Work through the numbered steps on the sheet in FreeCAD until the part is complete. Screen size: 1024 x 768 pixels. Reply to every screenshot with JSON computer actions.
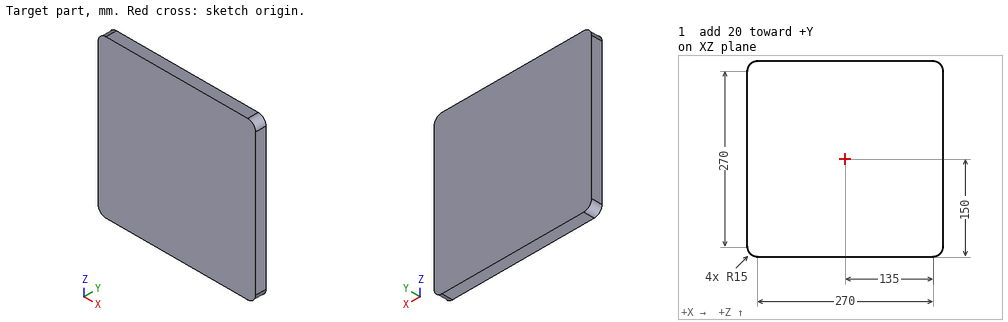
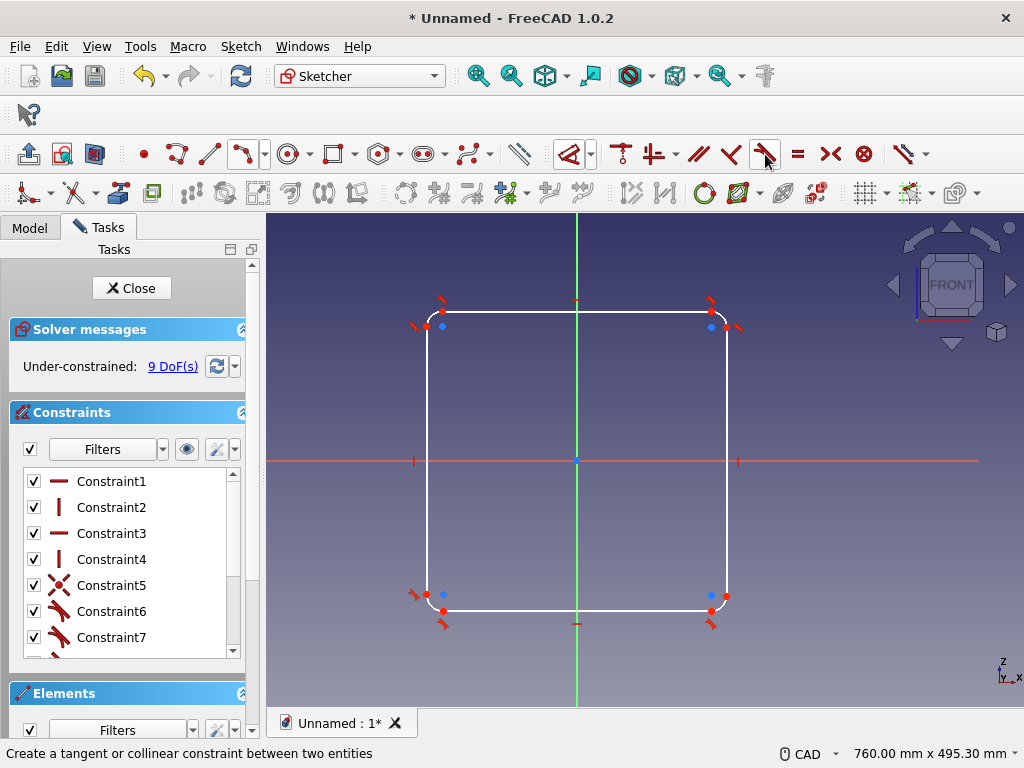
{"action": "left_click", "coordinate": [727, 408]}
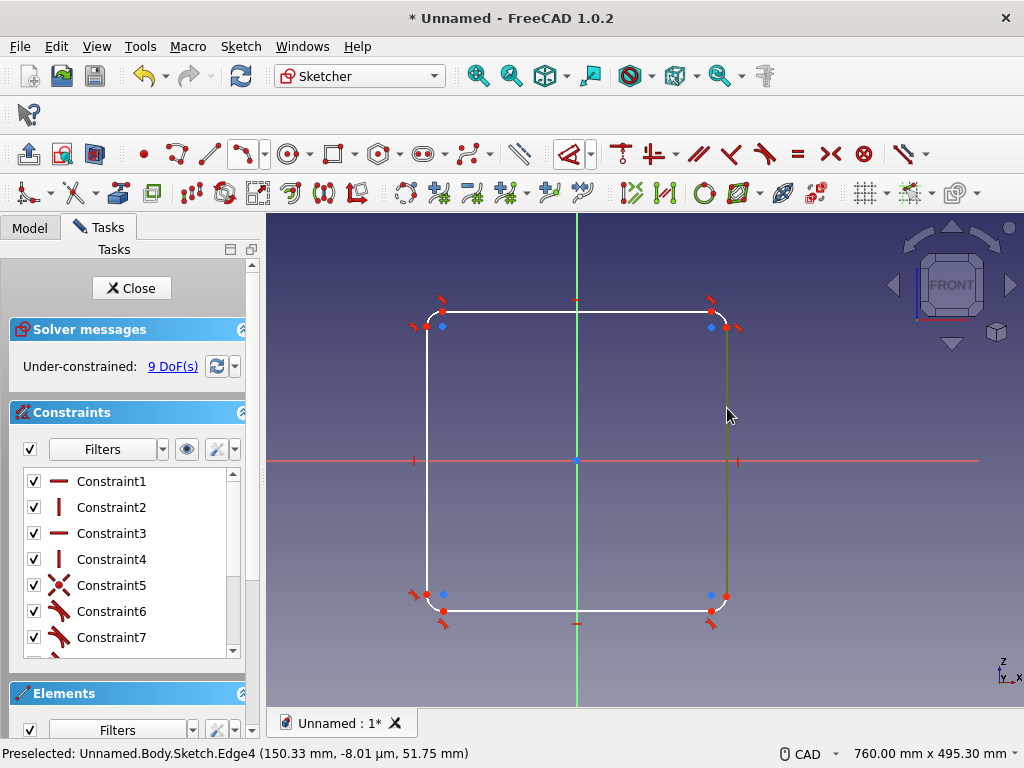
{"action": "left_click", "coordinate": [722, 607]}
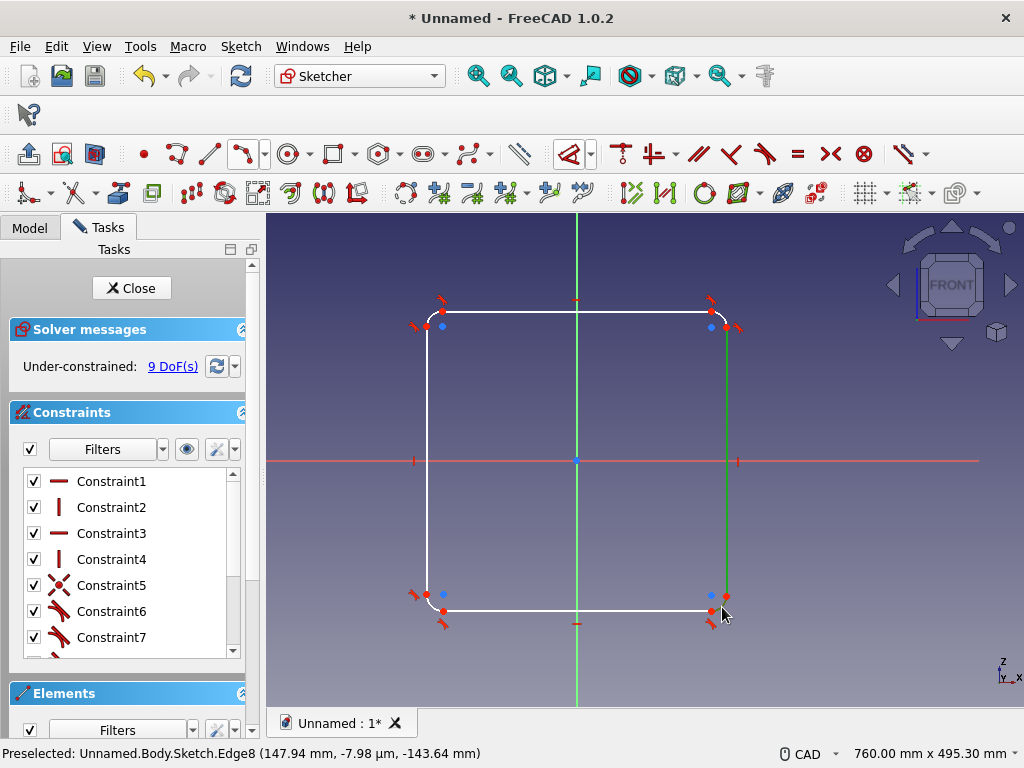
{"action": "left_click", "coordinate": [765, 154]}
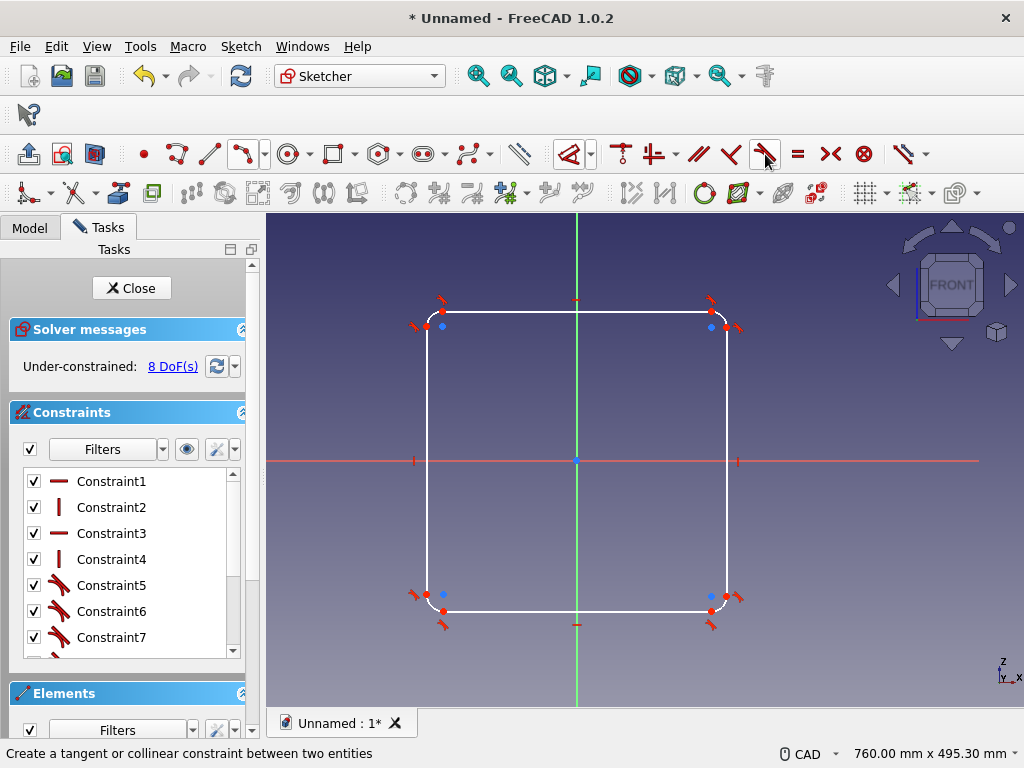
{"action": "left_click", "coordinate": [432, 607]}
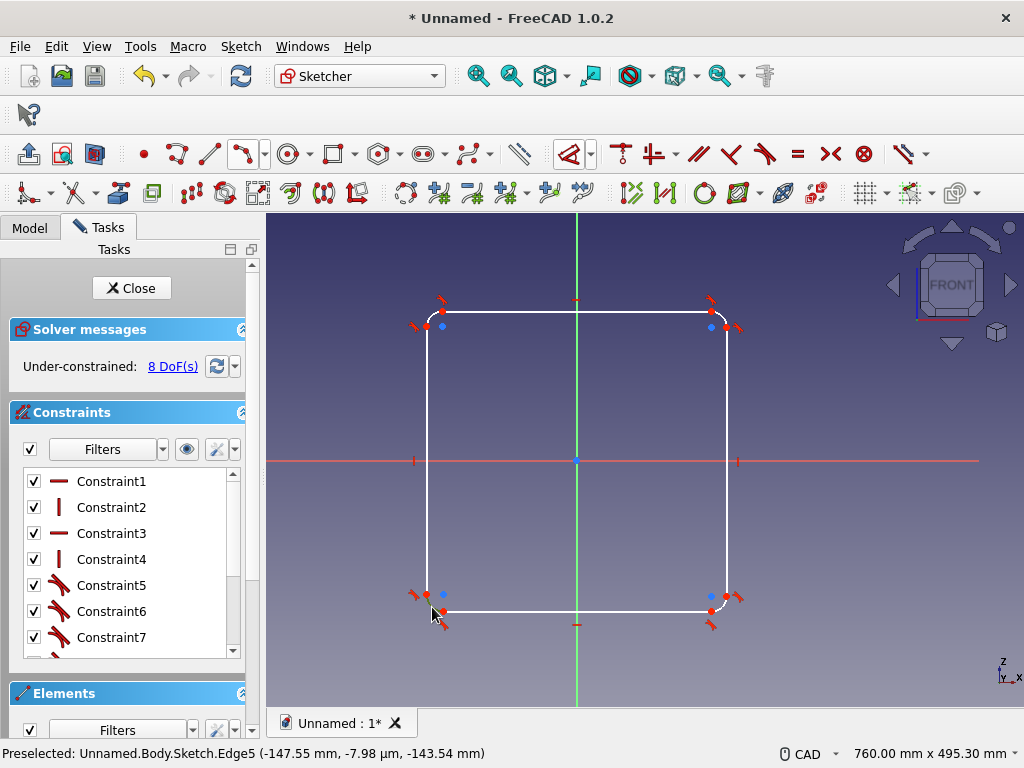
{"action": "left_click", "coordinate": [431, 316]}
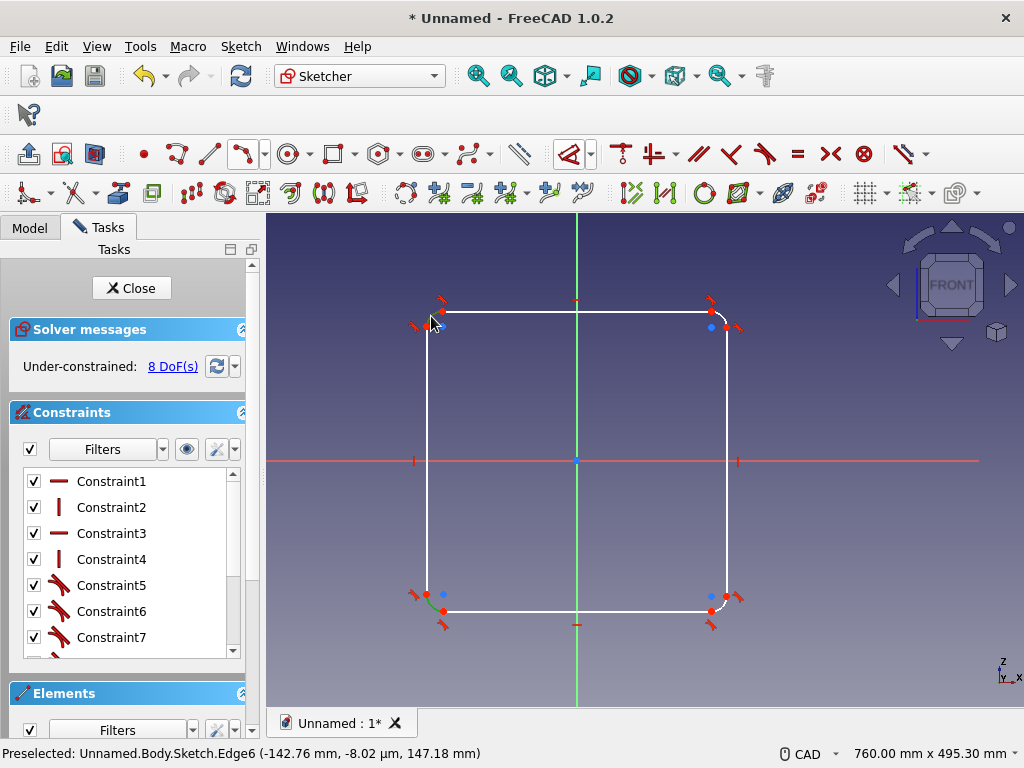
{"action": "left_click", "coordinate": [722, 316]}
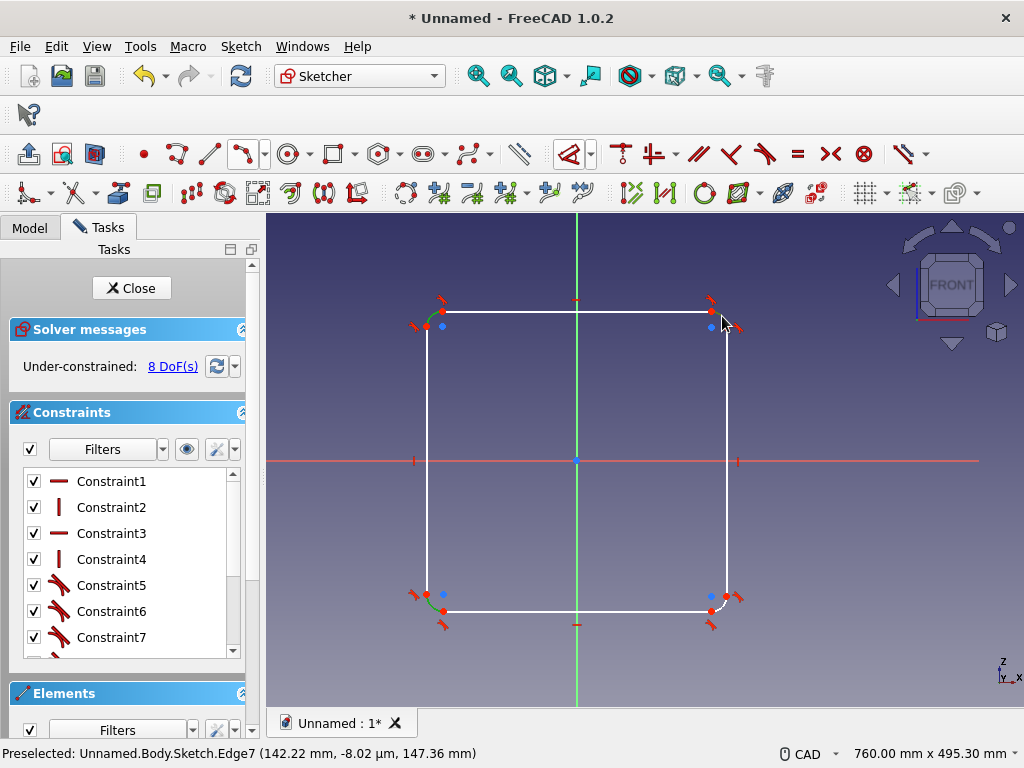
{"action": "left_click", "coordinate": [722, 607]}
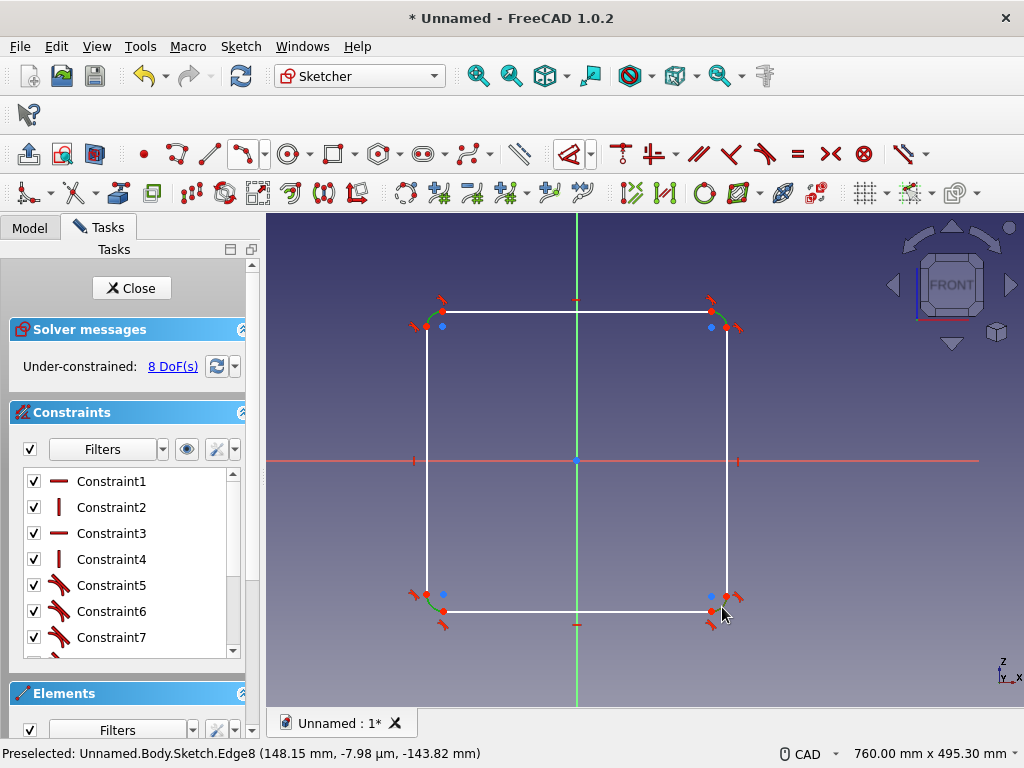
{"action": "left_click", "coordinate": [798, 154]}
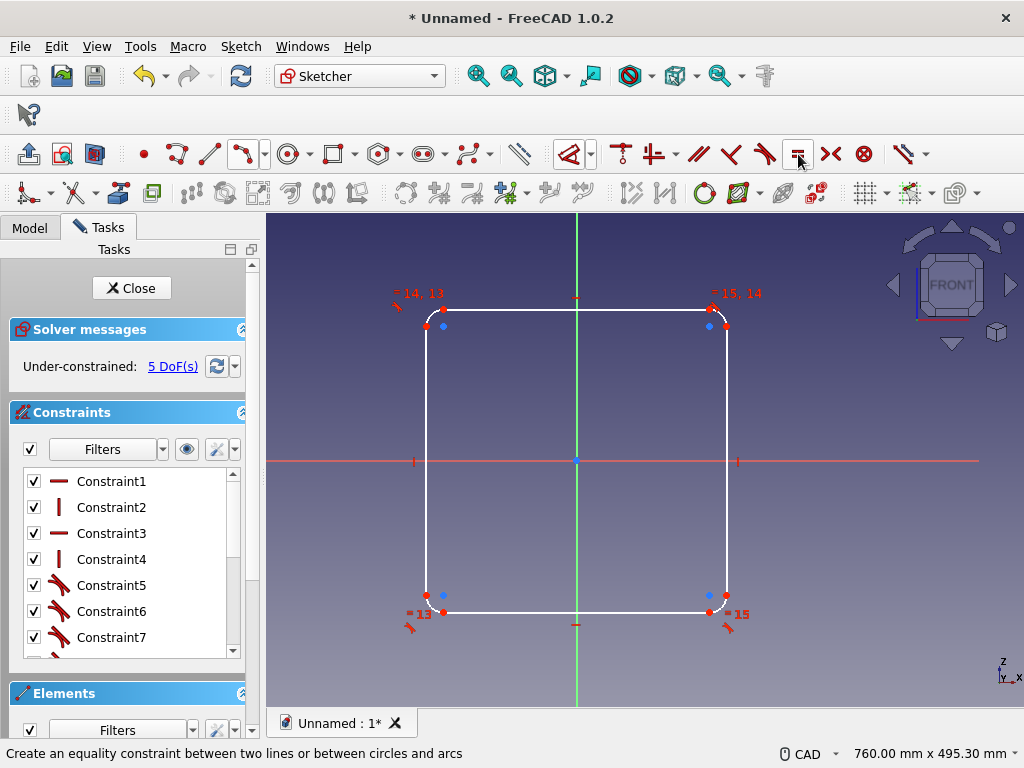
{"action": "left_click", "coordinate": [568, 154]}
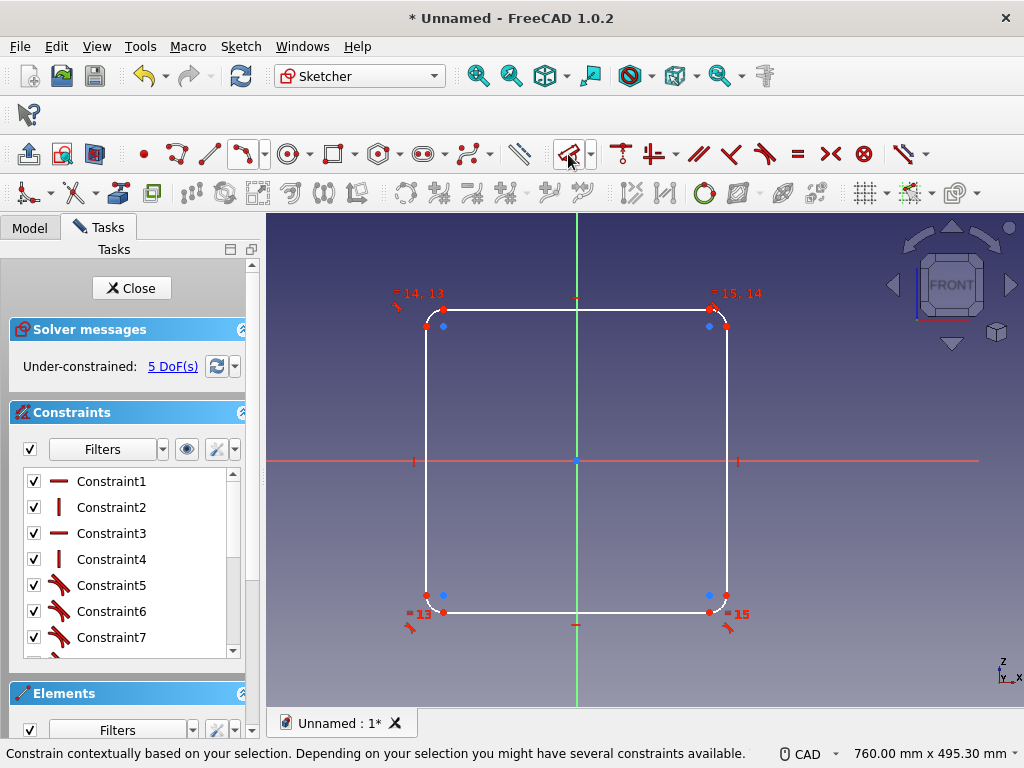
{"action": "scroll", "coordinate": [431, 608], "scroll_direction": "up", "scroll_amount": 5}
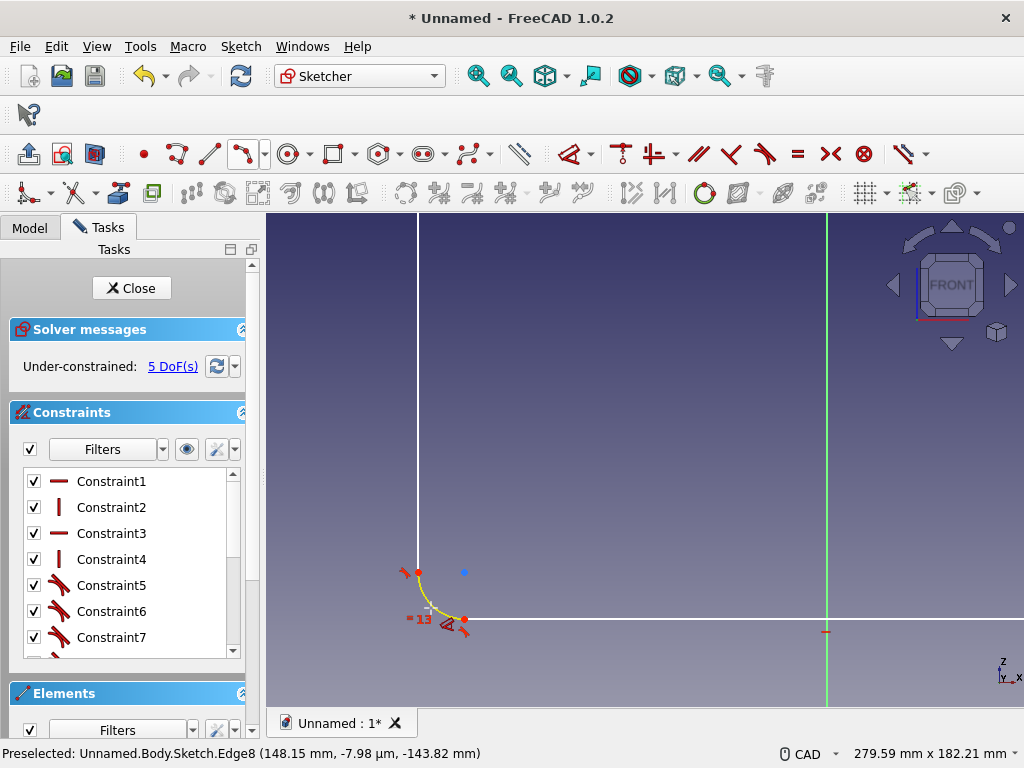
{"action": "left_click", "coordinate": [432, 605]}
{"action": "left_click", "coordinate": [409, 627]}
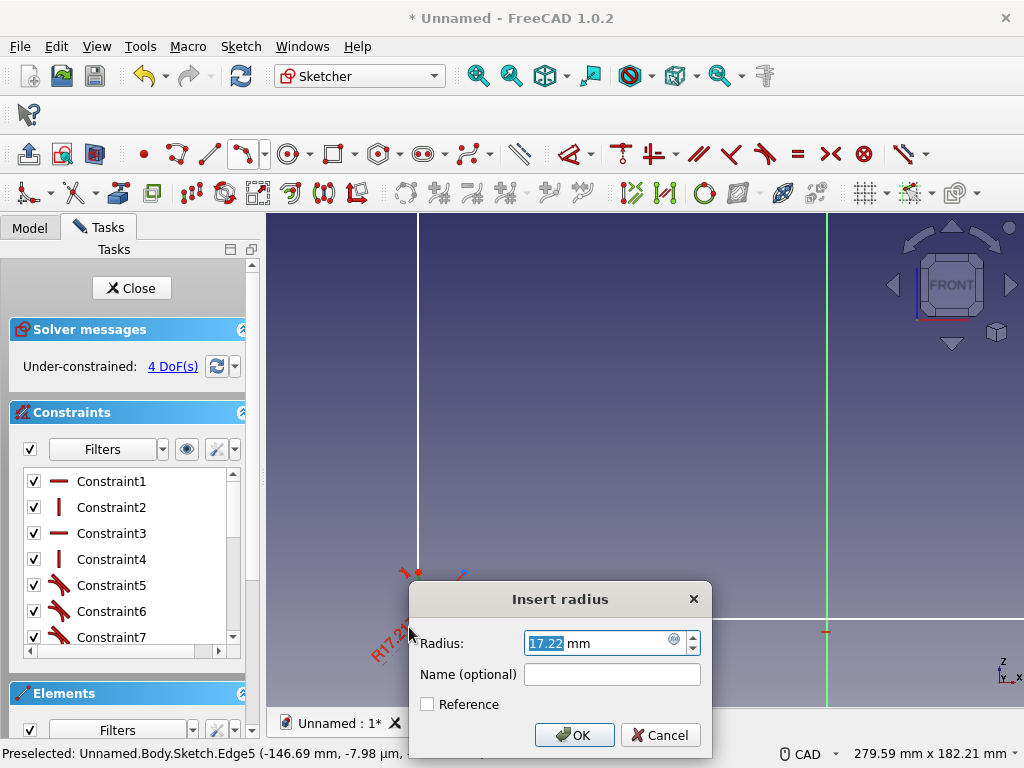
{"action": "type", "text": "15"}
{"action": "key", "text": "Return"}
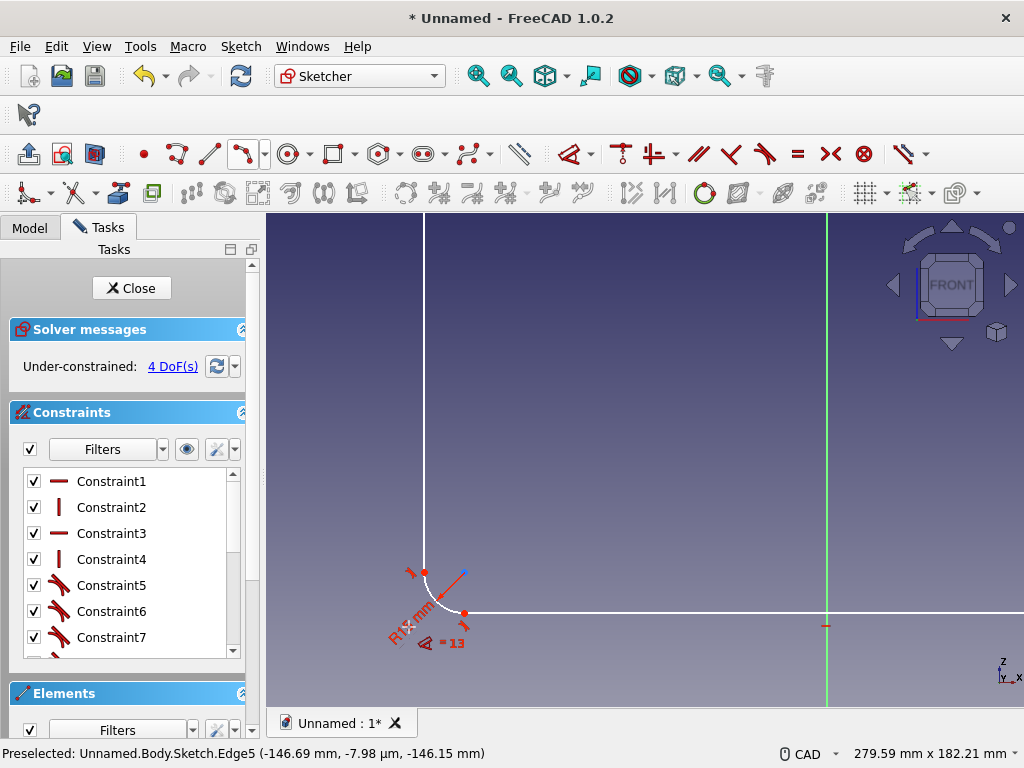
{"action": "left_click", "coordinate": [682, 613]}
{"action": "left_click", "coordinate": [662, 647]}